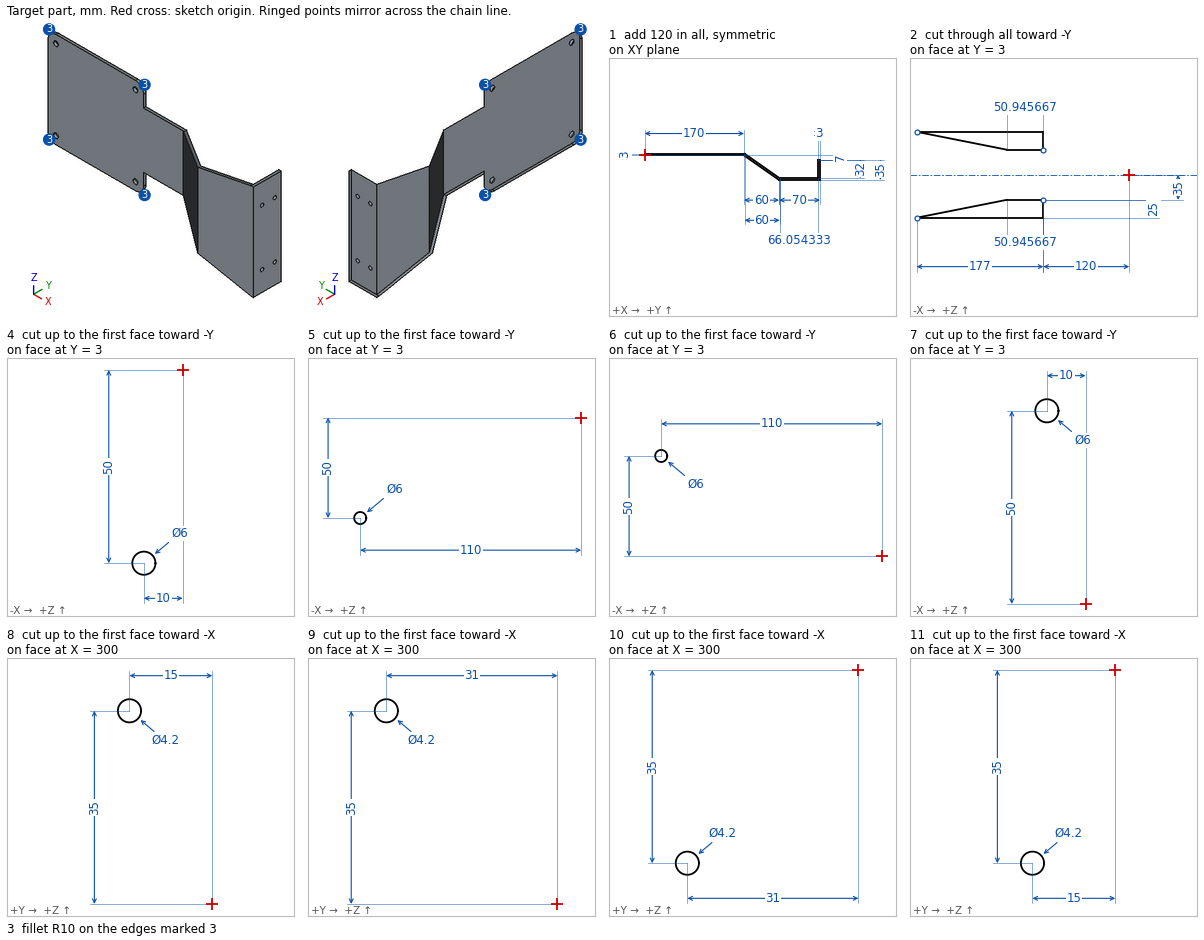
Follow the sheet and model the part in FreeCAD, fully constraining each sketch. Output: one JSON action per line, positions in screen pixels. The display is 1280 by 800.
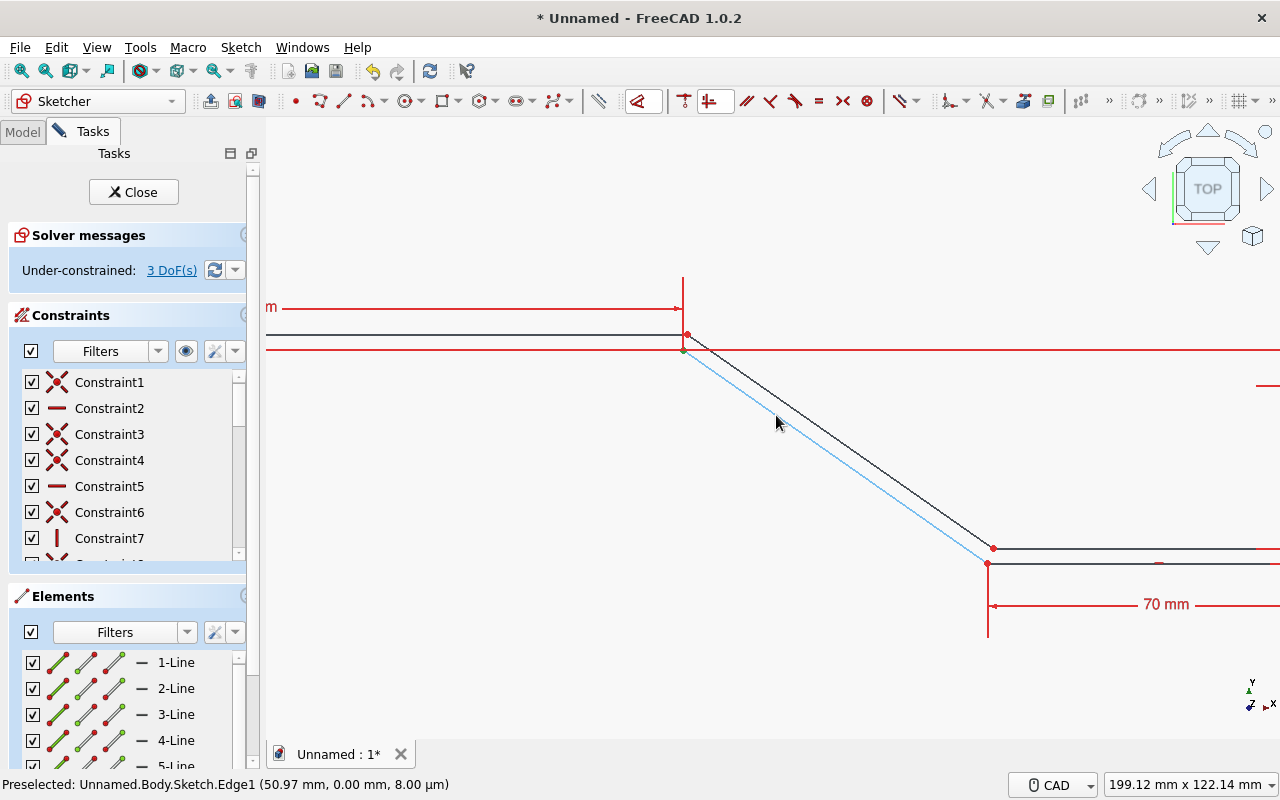
{"action": "left_click", "coordinate": [775, 414]}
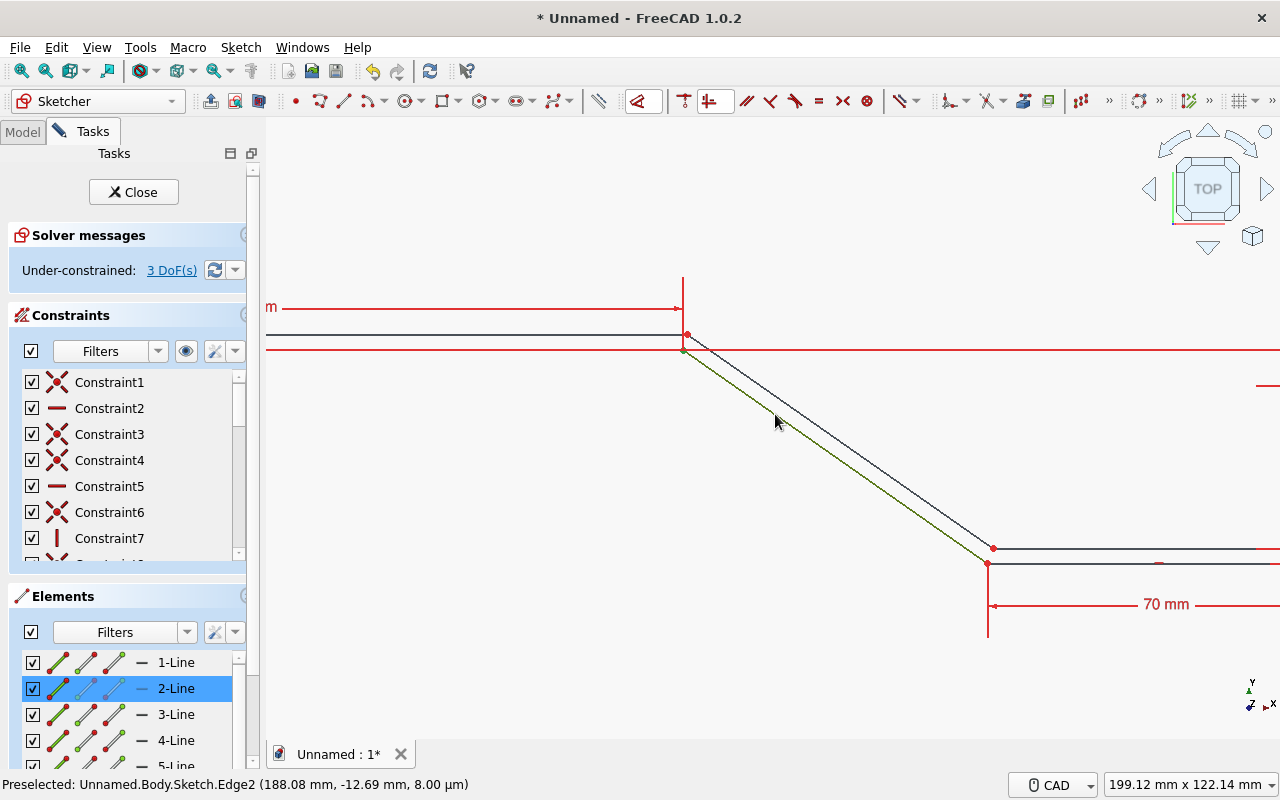
{"action": "left_click", "coordinate": [656, 102]}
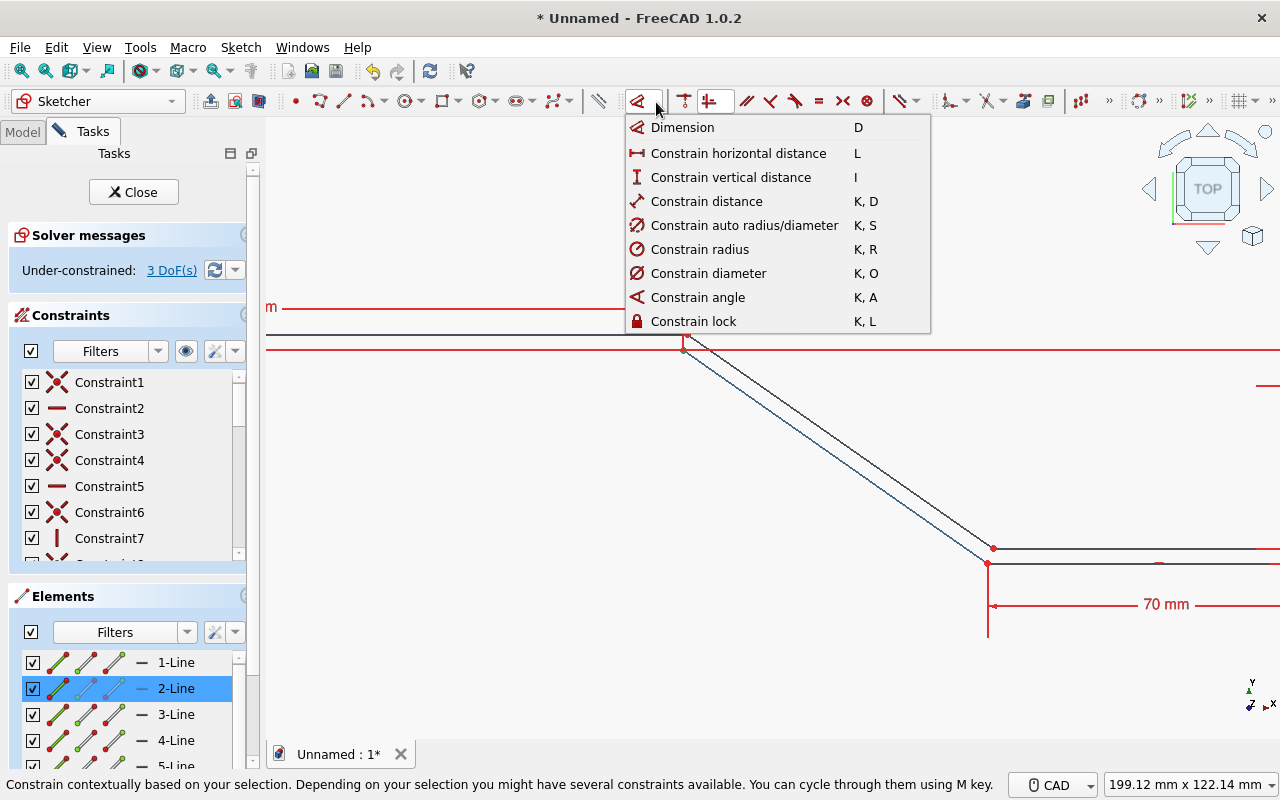
{"action": "left_click", "coordinate": [778, 153]}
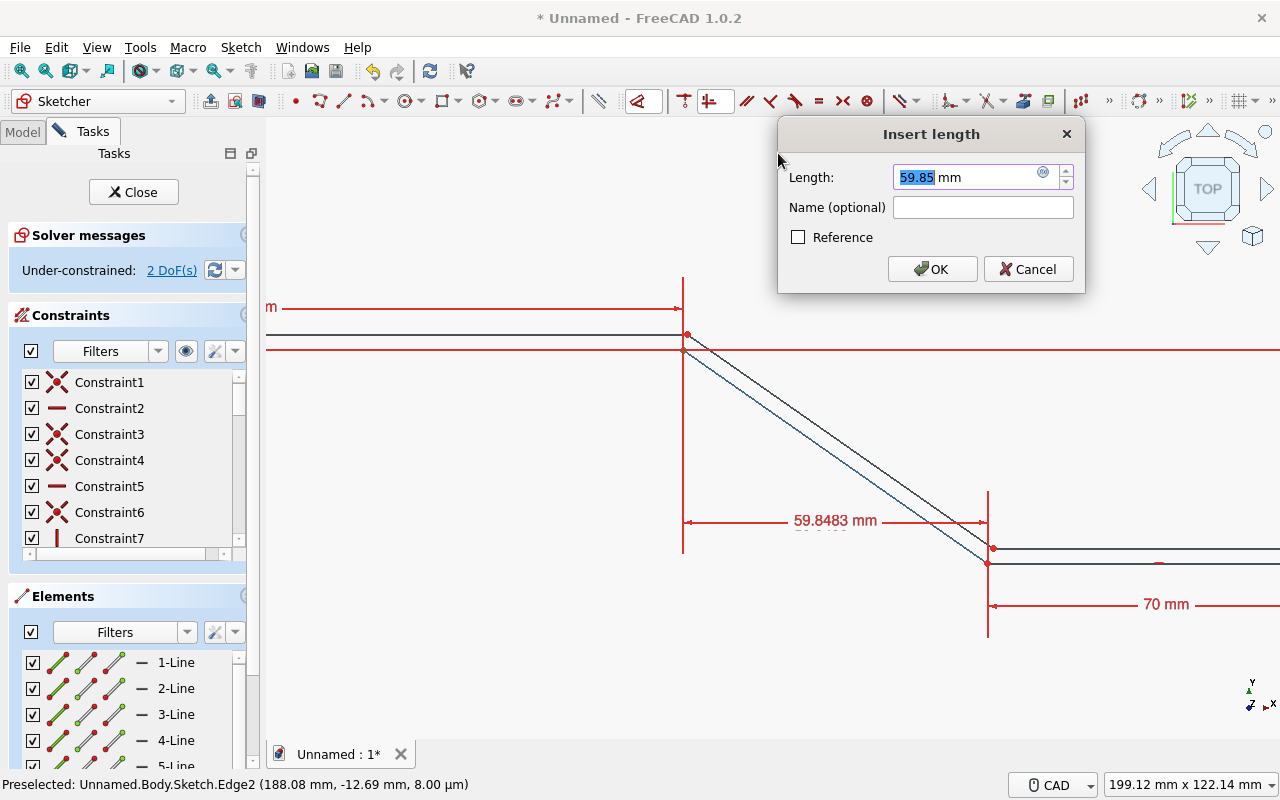
{"action": "type", "text": "60"}
{"action": "key", "text": "Return"}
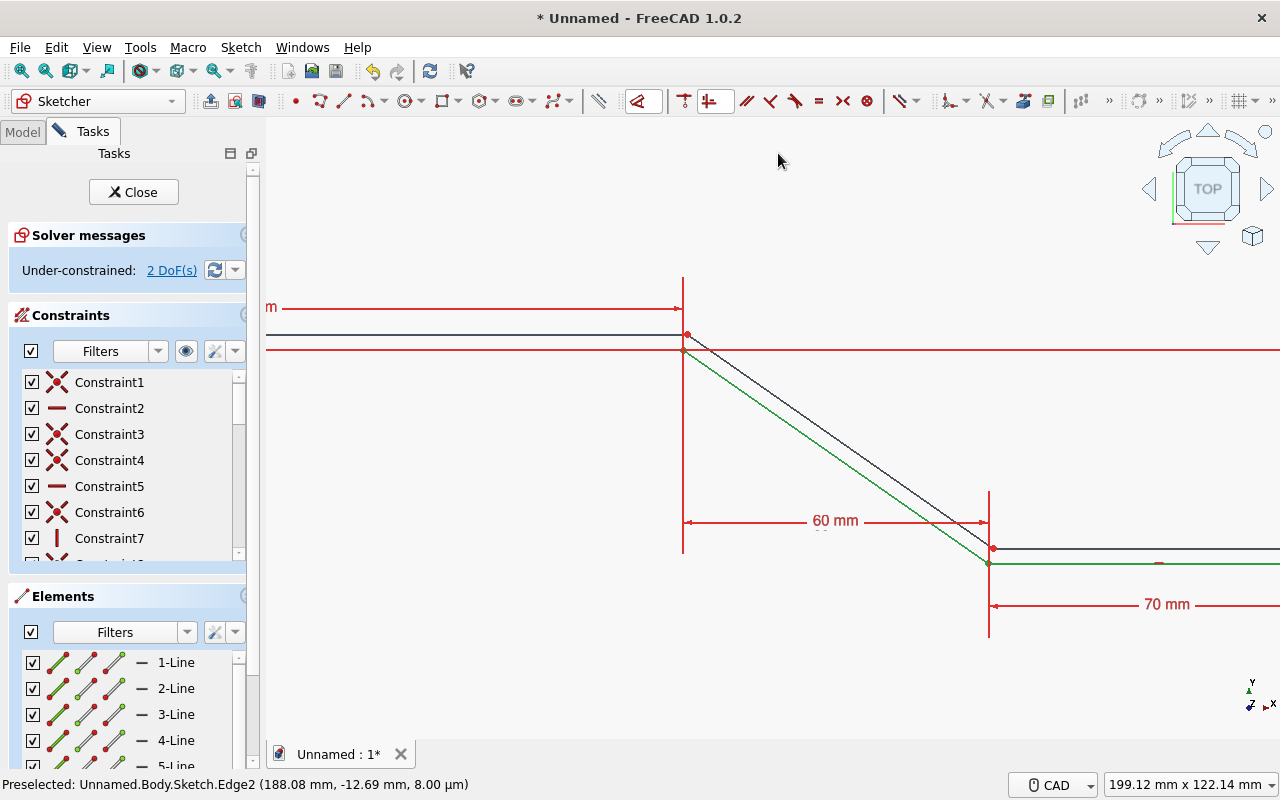
{"action": "left_click", "coordinate": [901, 485]}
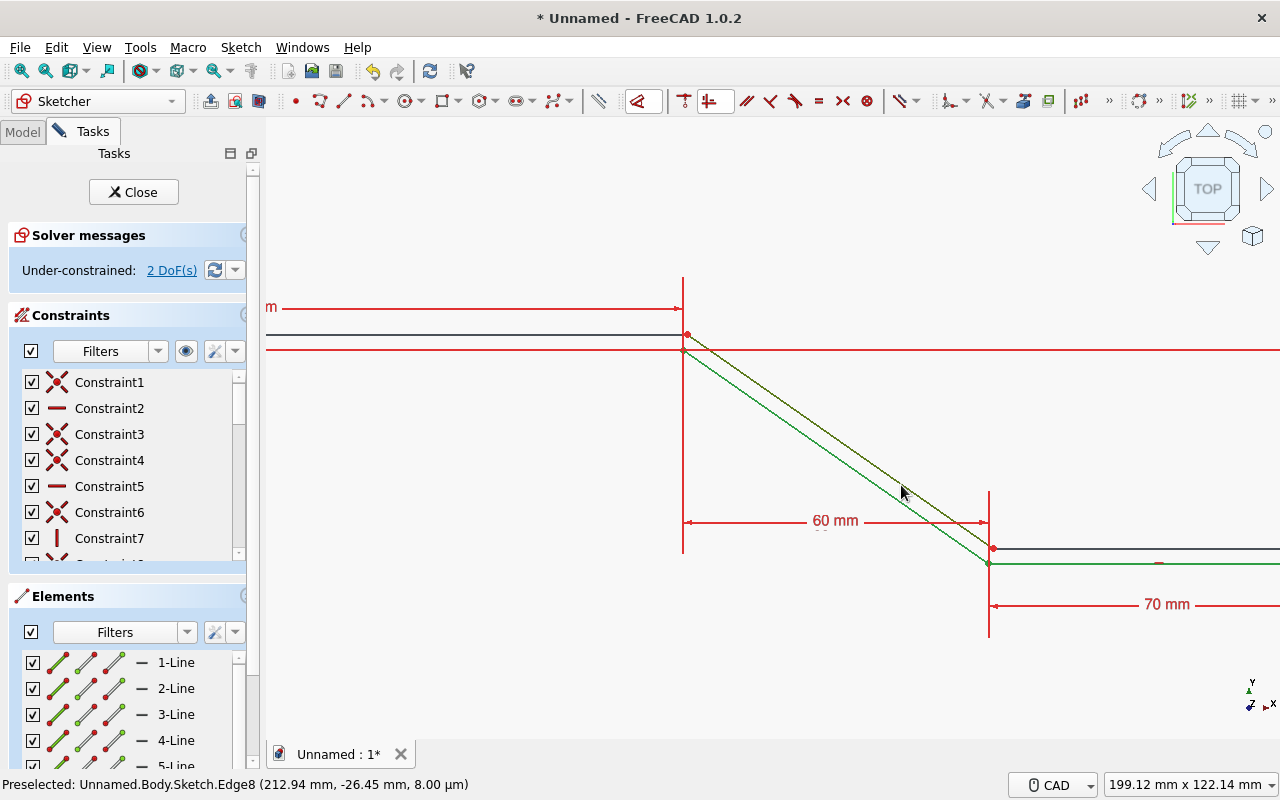
{"action": "key", "text": "l"}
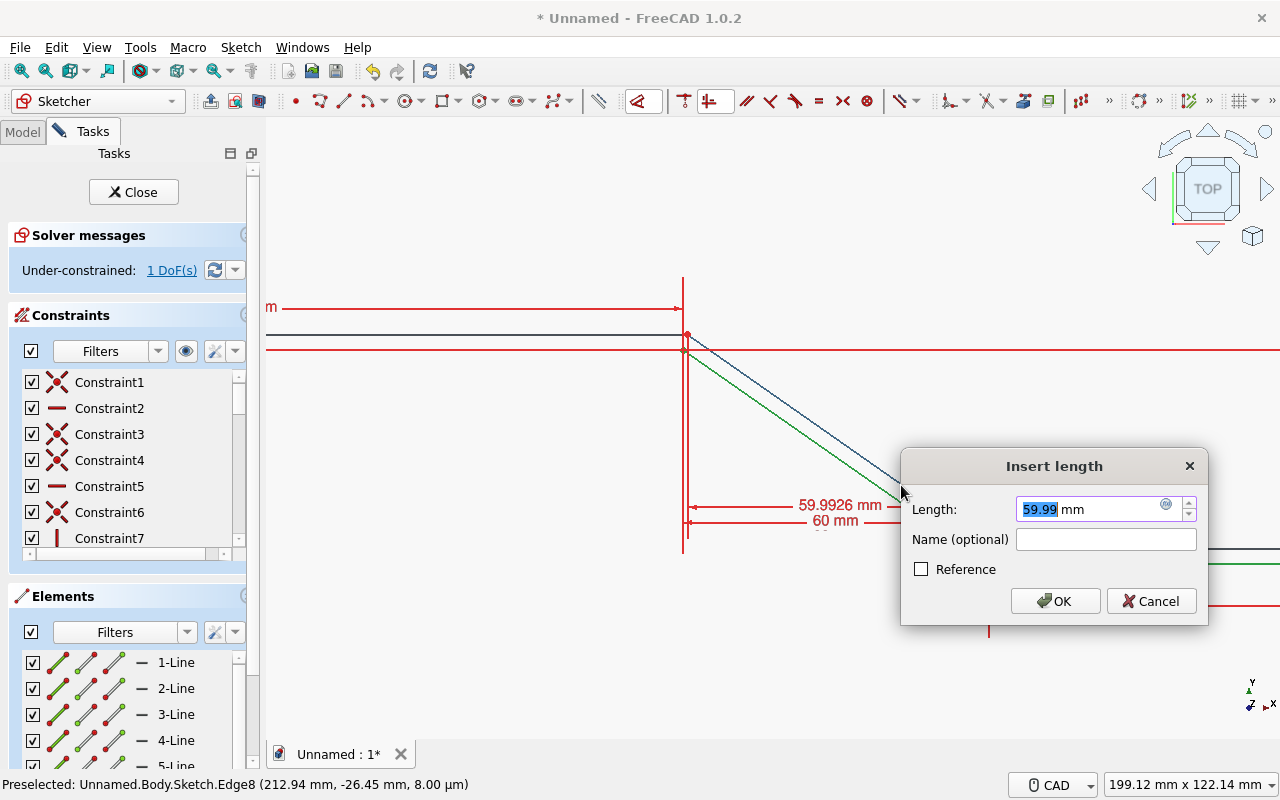
{"action": "type", "text": "60"}
{"action": "key", "text": "Return"}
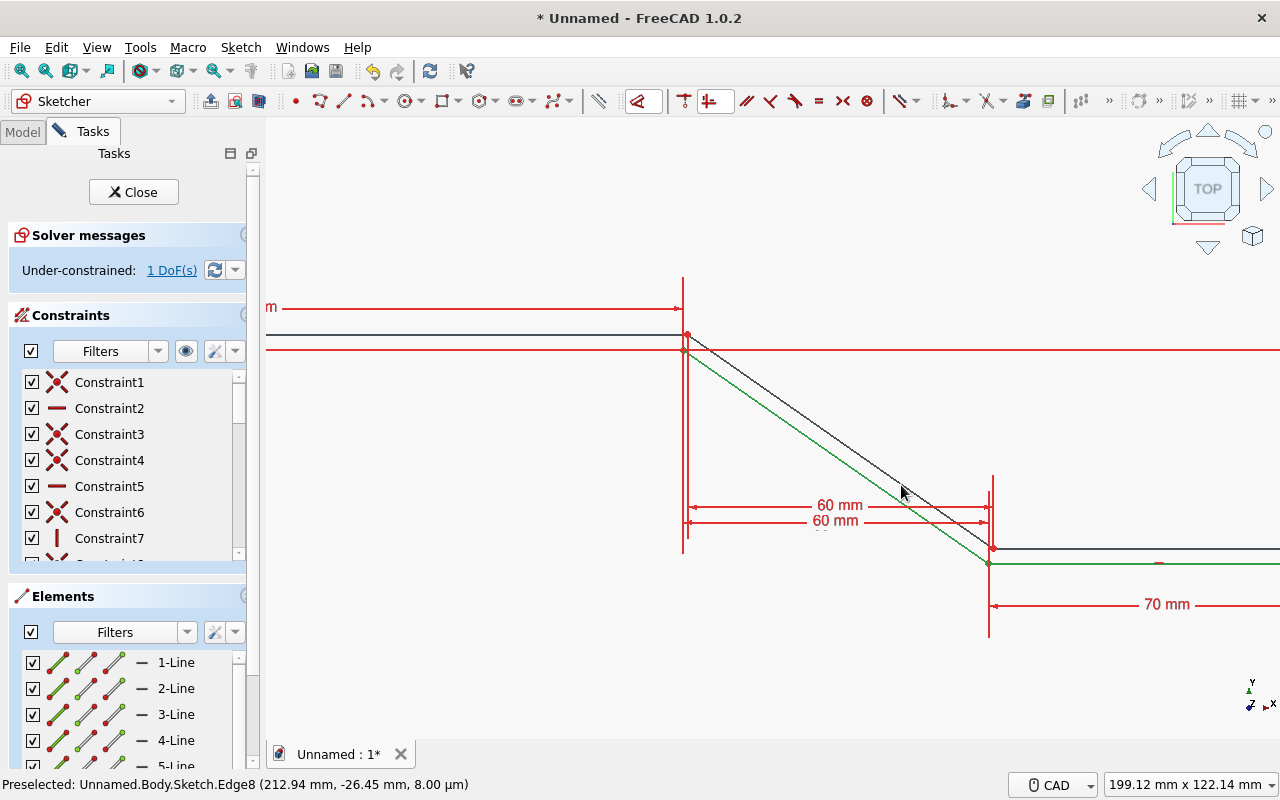
{"action": "left_click", "coordinate": [1094, 549]}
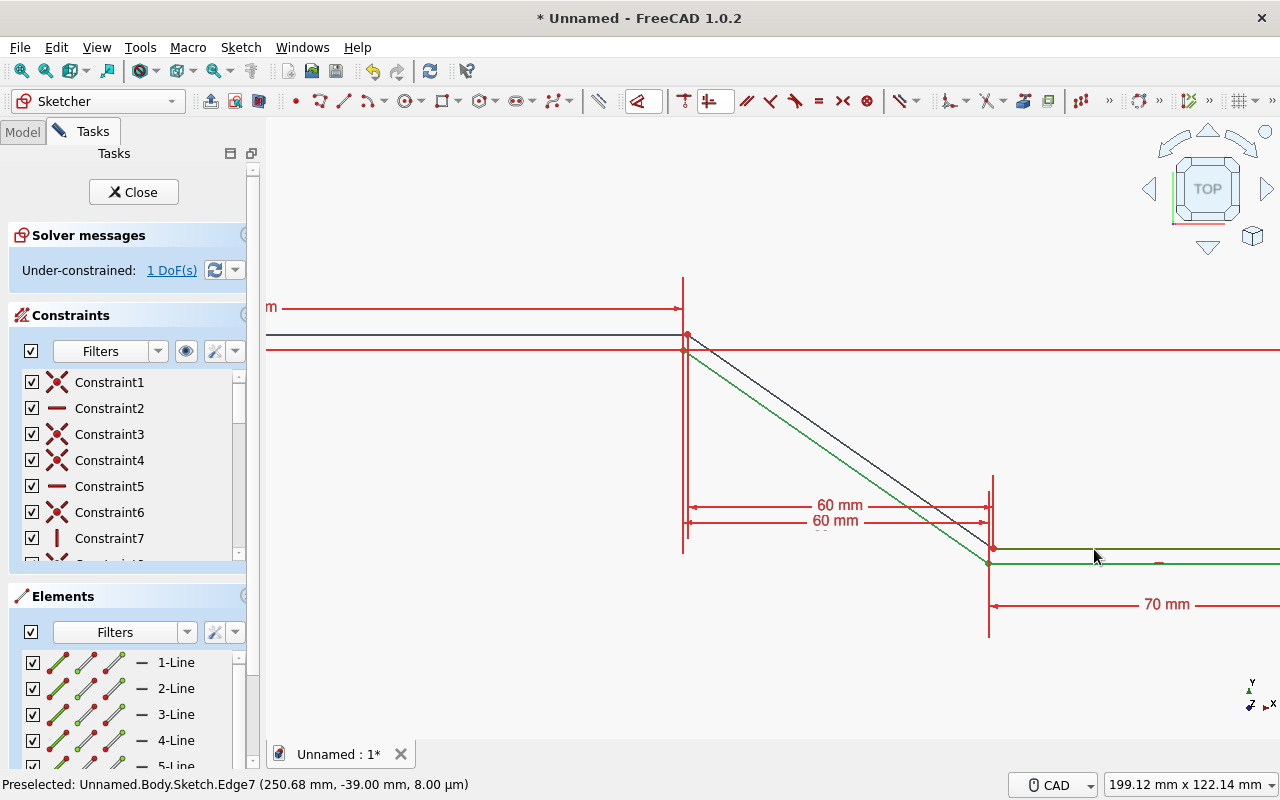
{"action": "left_click", "coordinate": [656, 102]}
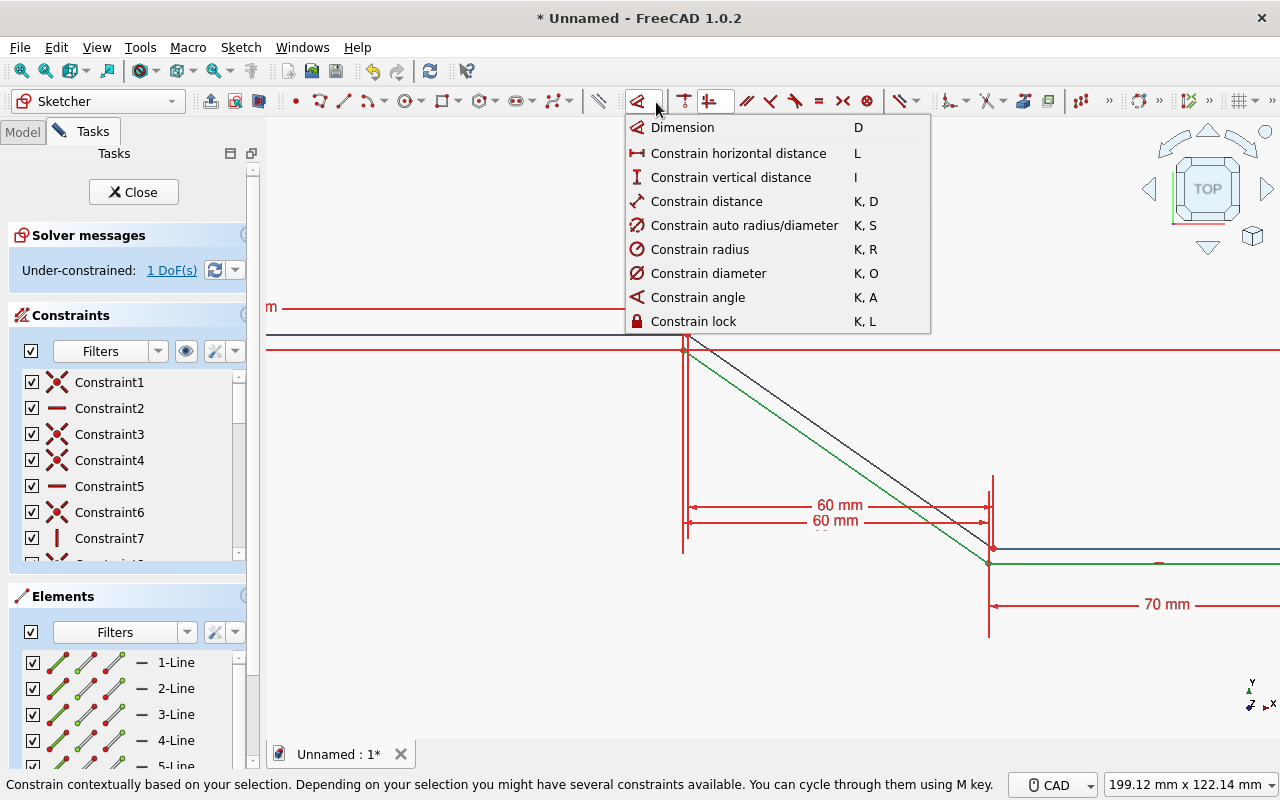
{"action": "left_click", "coordinate": [778, 153]}